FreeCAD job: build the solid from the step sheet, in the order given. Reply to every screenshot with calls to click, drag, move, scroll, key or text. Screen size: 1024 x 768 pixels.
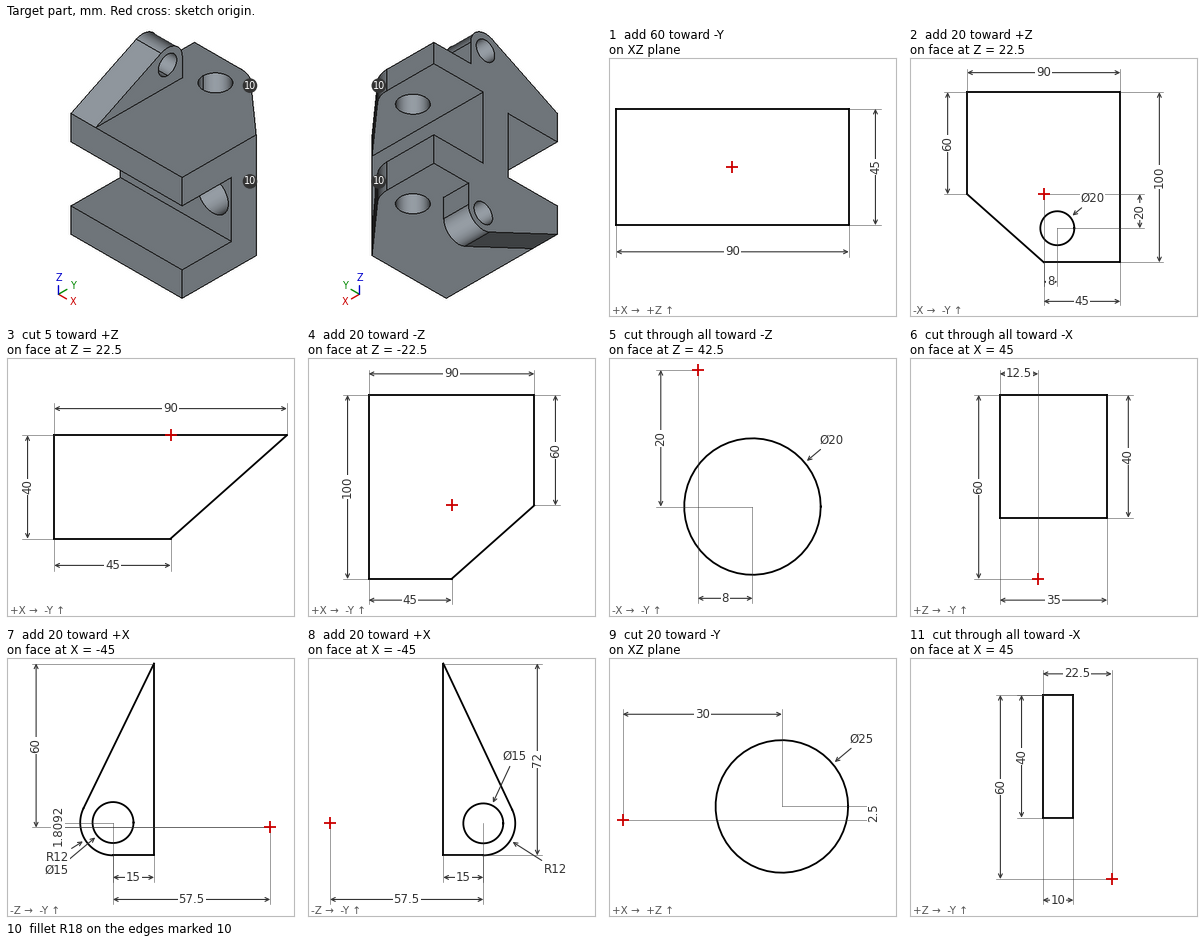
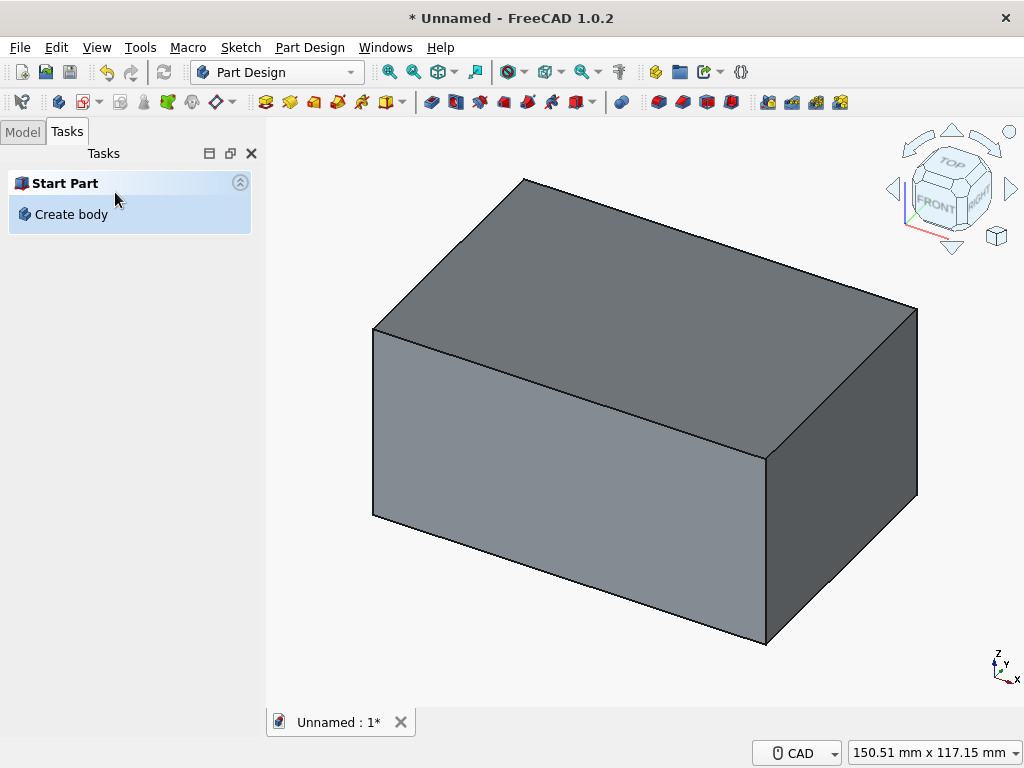
click(701, 337)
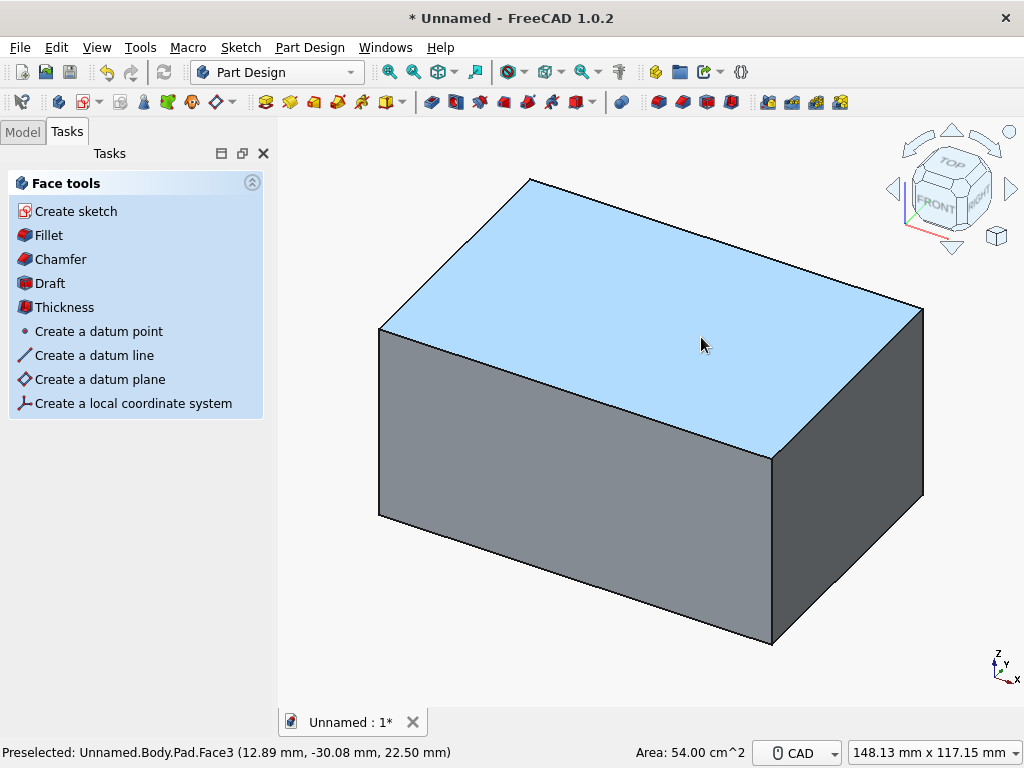
click(84, 102)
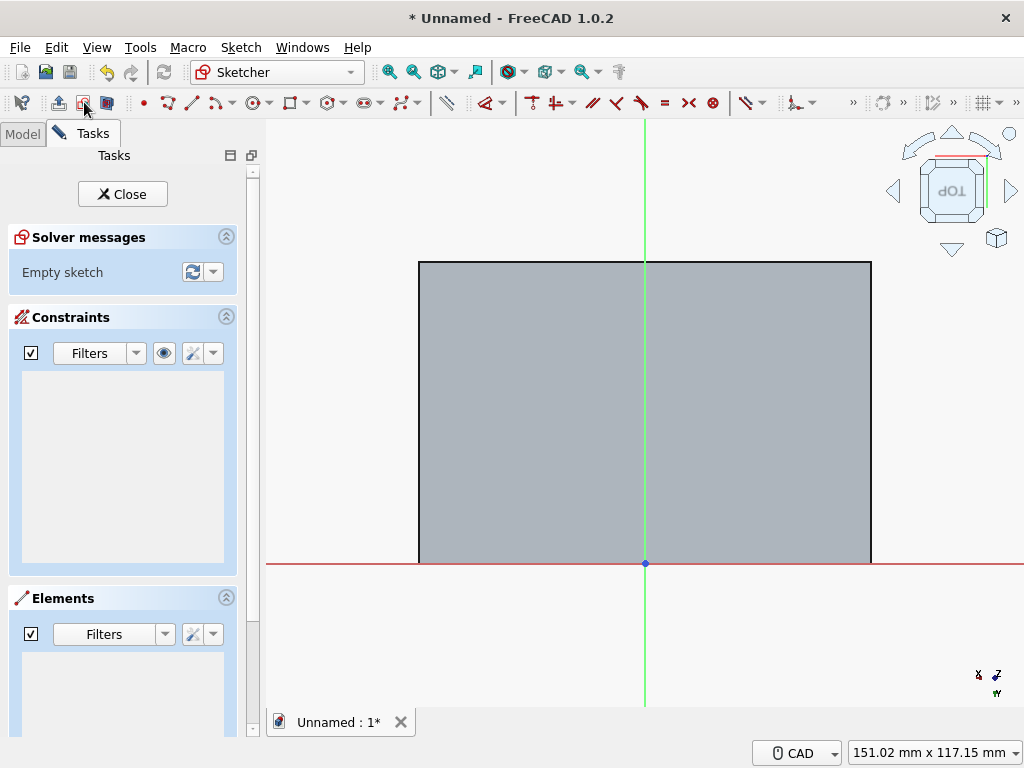
scroll(294, 147, down, 1)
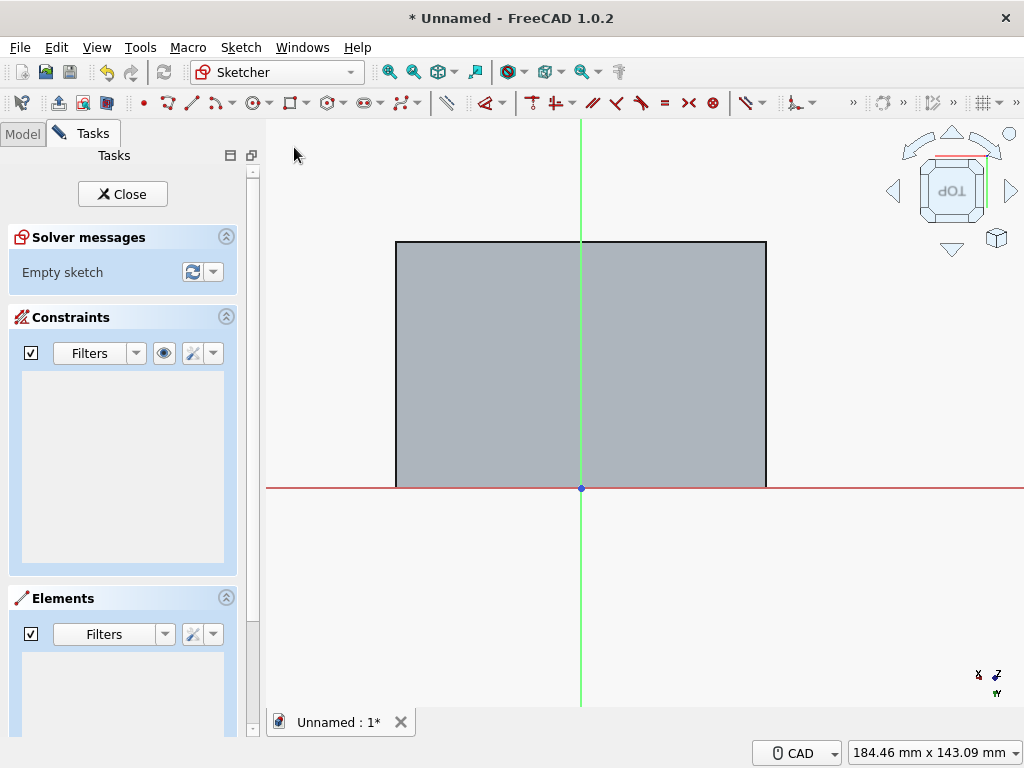
click(168, 104)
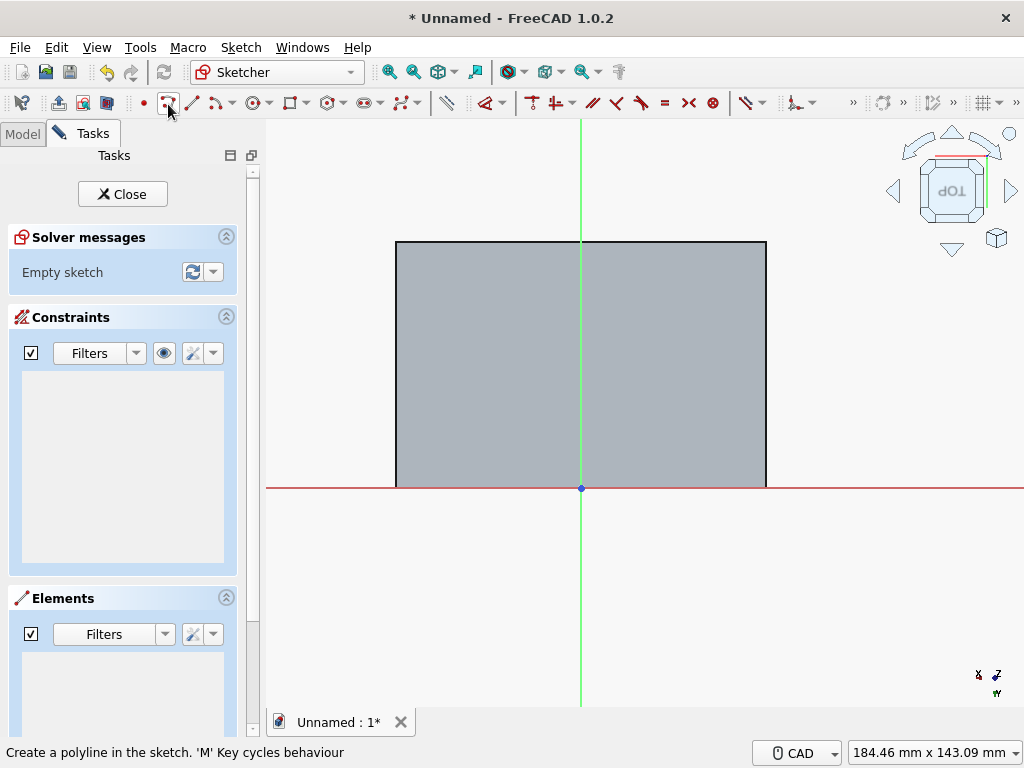
click(581, 652)
click(766, 652)
click(766, 242)
click(396, 242)
click(396, 488)
click(581, 653)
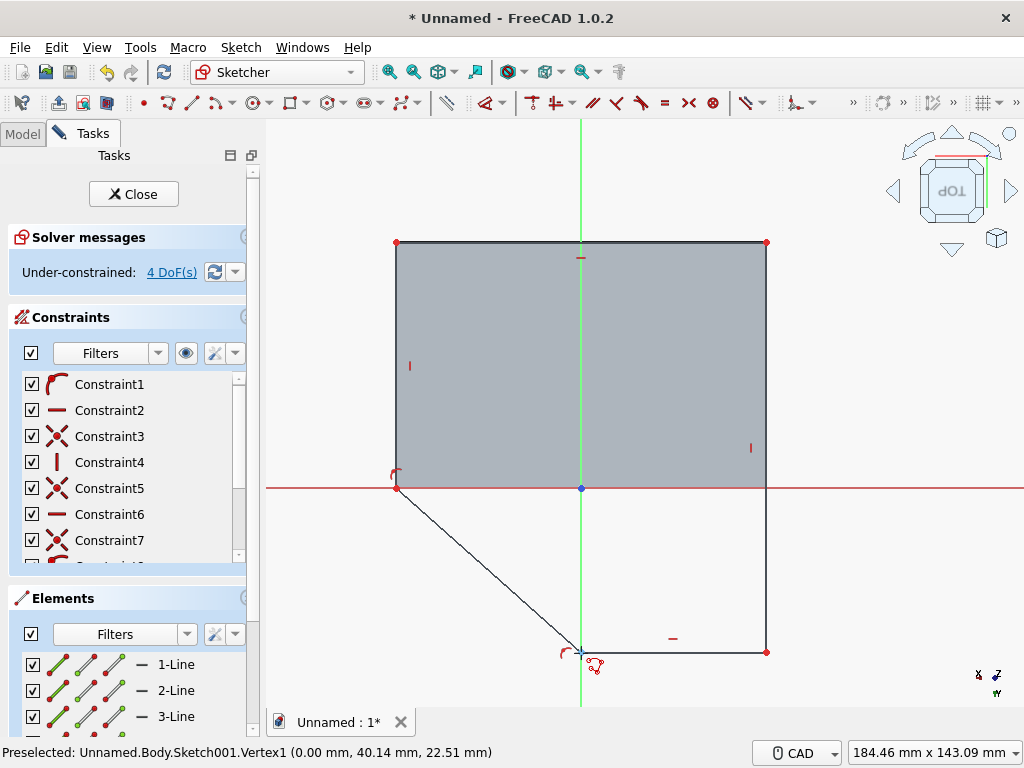
key(g)
key(c)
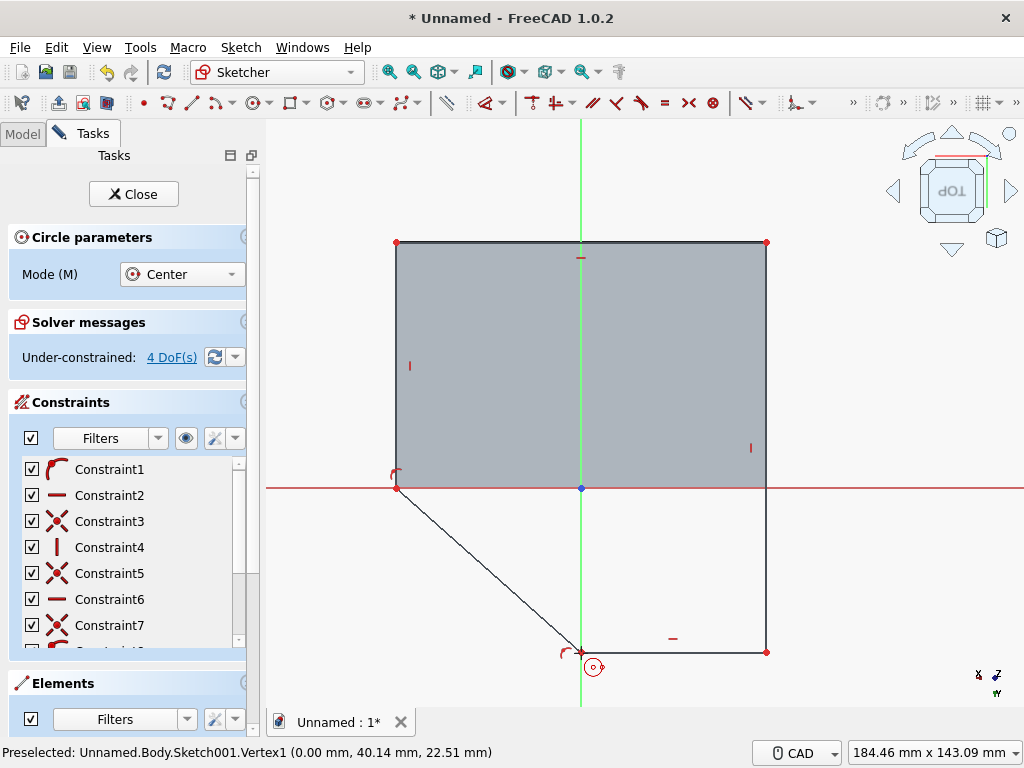
click(614, 570)
move(643, 541)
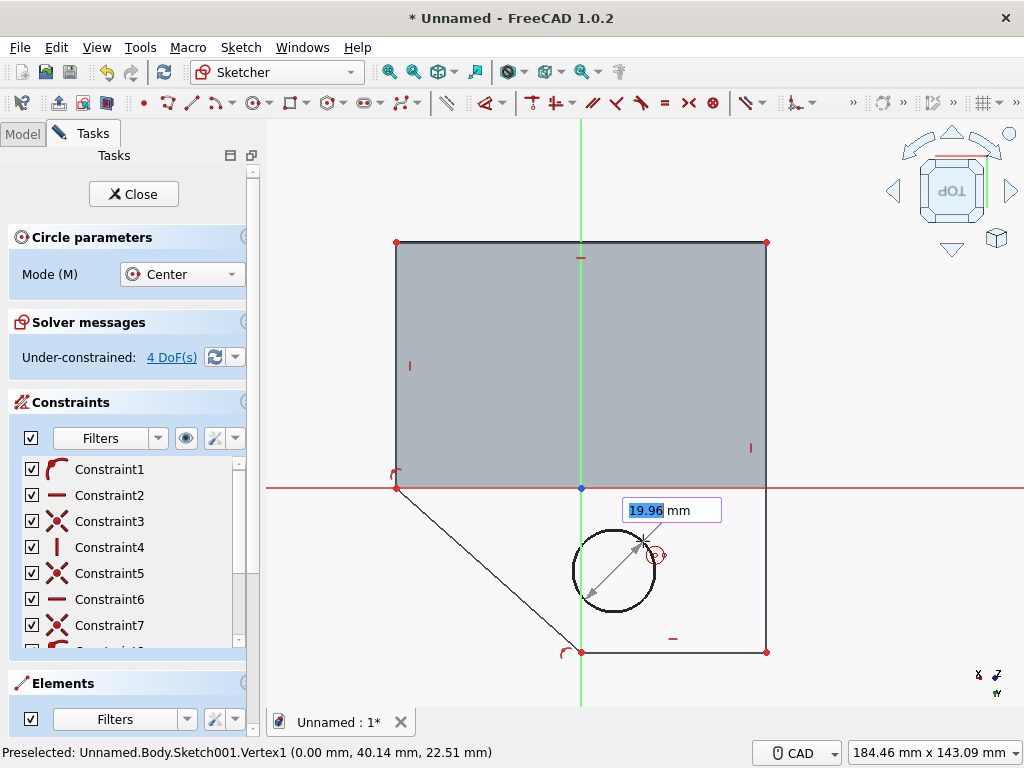
text(20)
key(Return)
key(Escape)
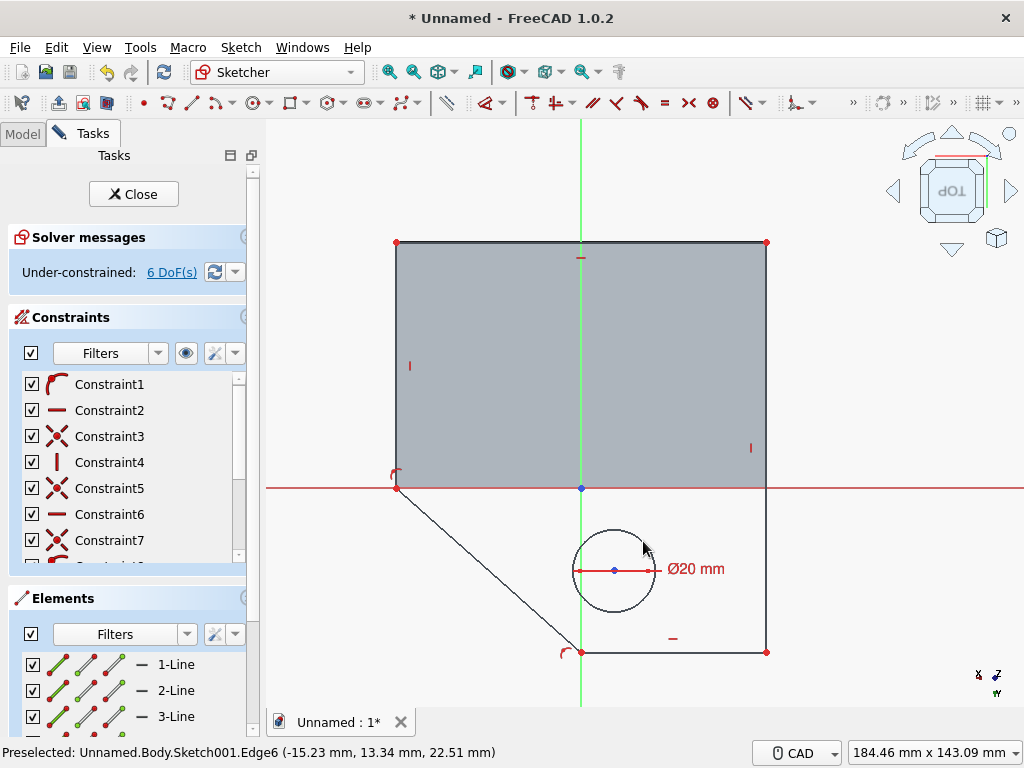
click(614, 571)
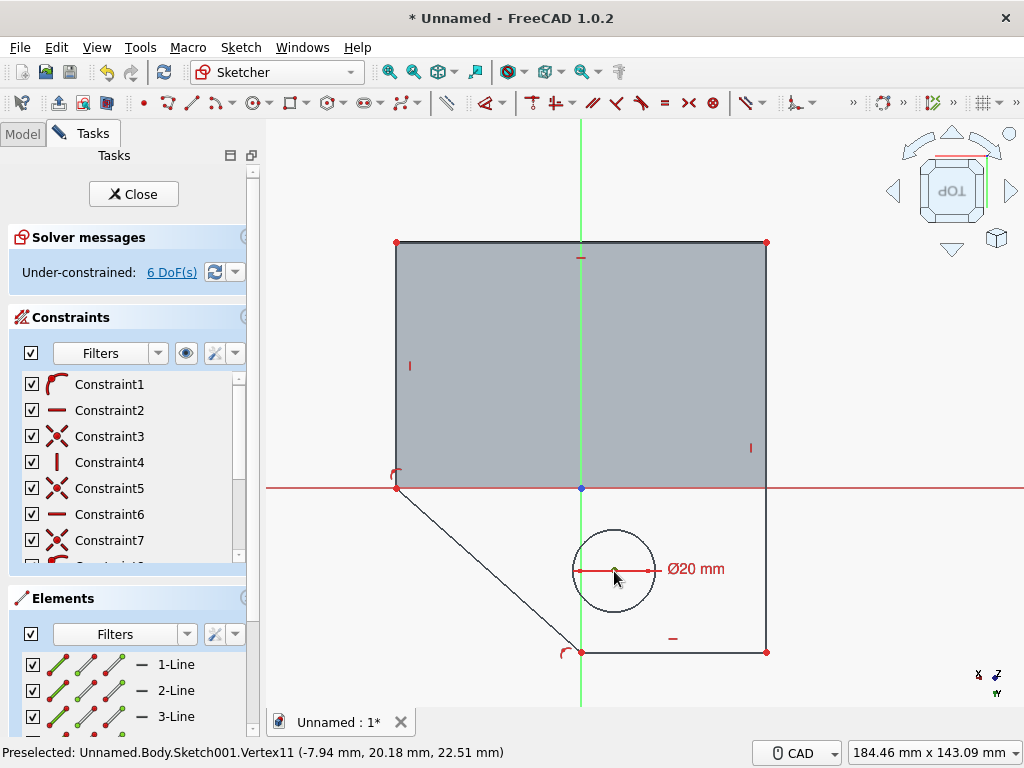
click(504, 104)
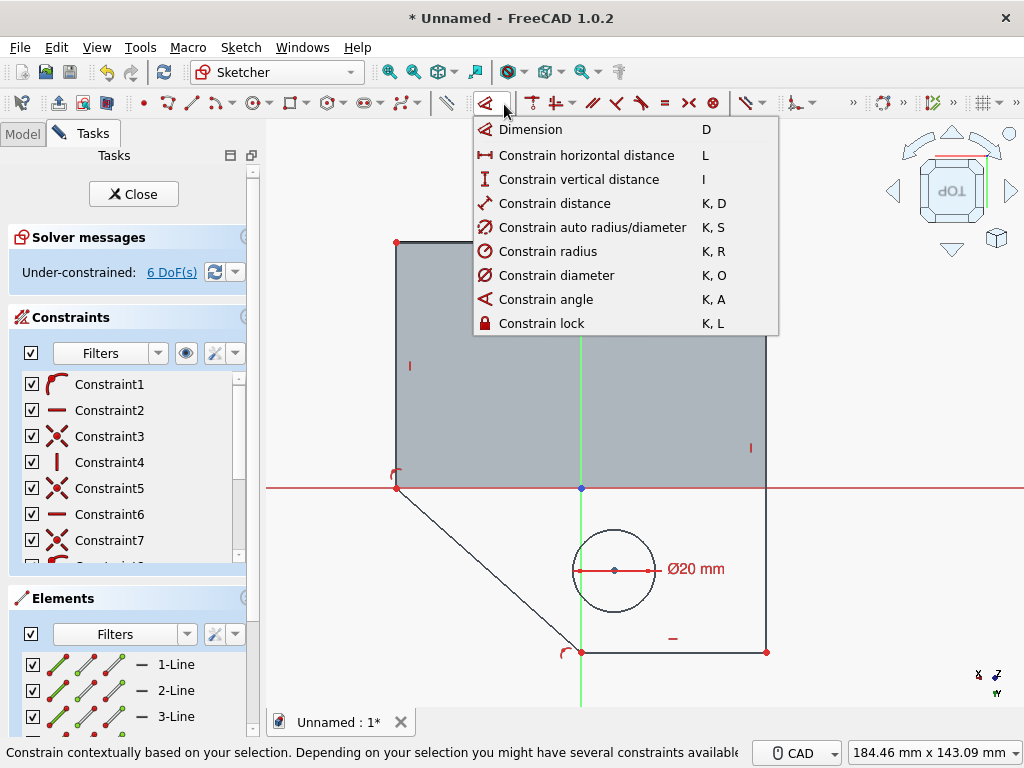
click(626, 155)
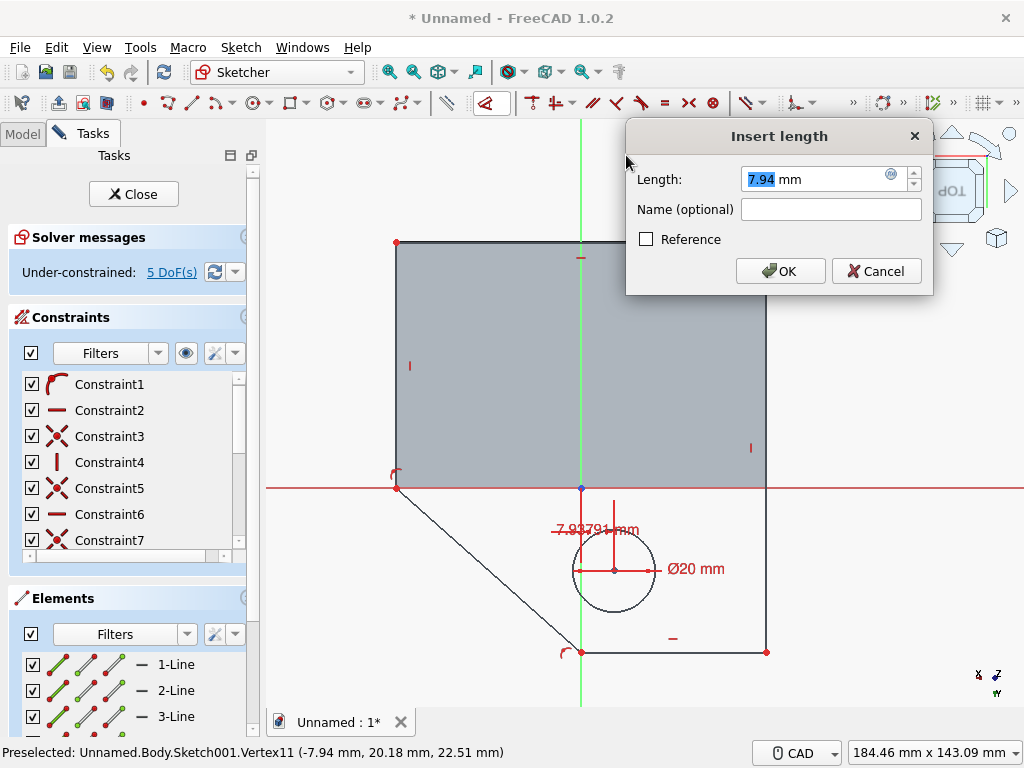
text(8)
key(Return)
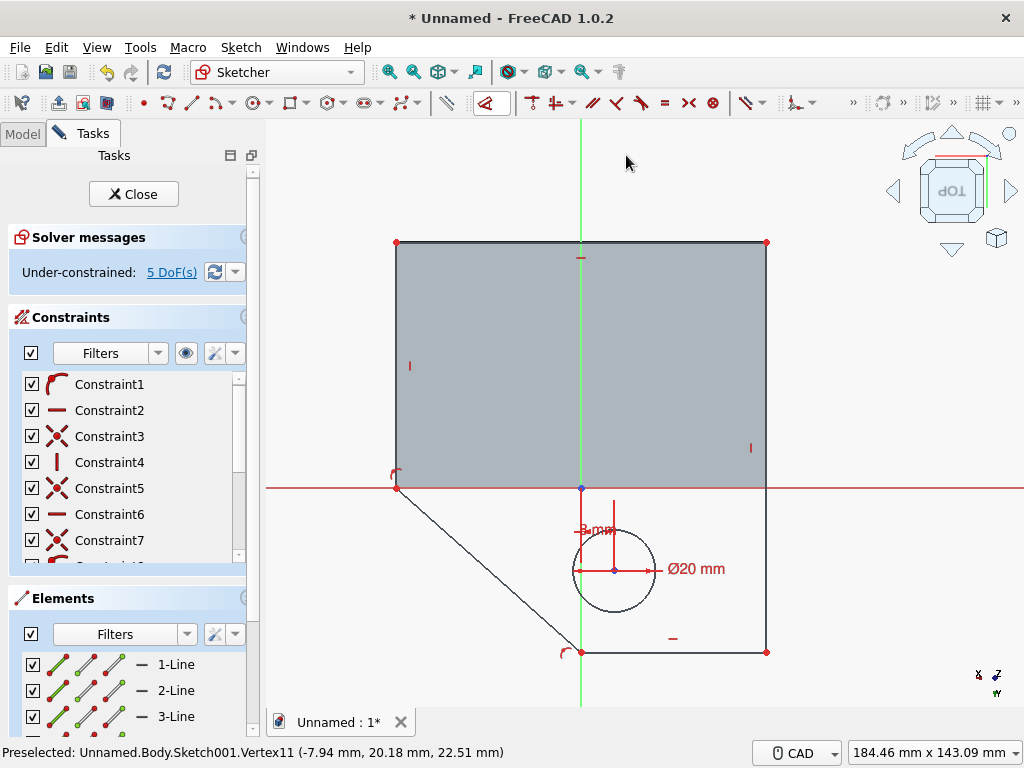
click(637, 653)